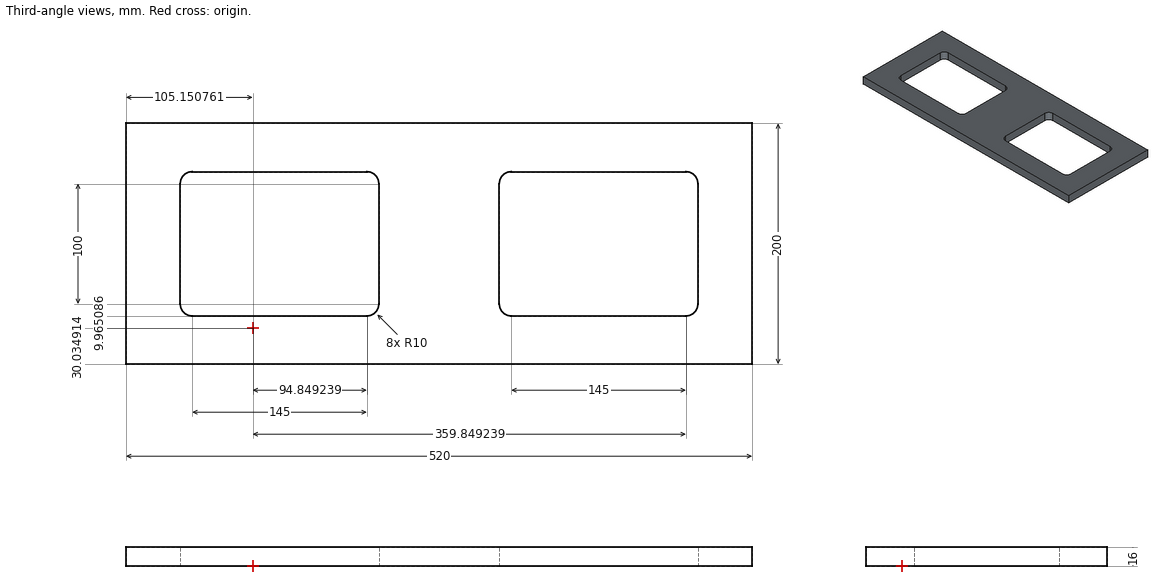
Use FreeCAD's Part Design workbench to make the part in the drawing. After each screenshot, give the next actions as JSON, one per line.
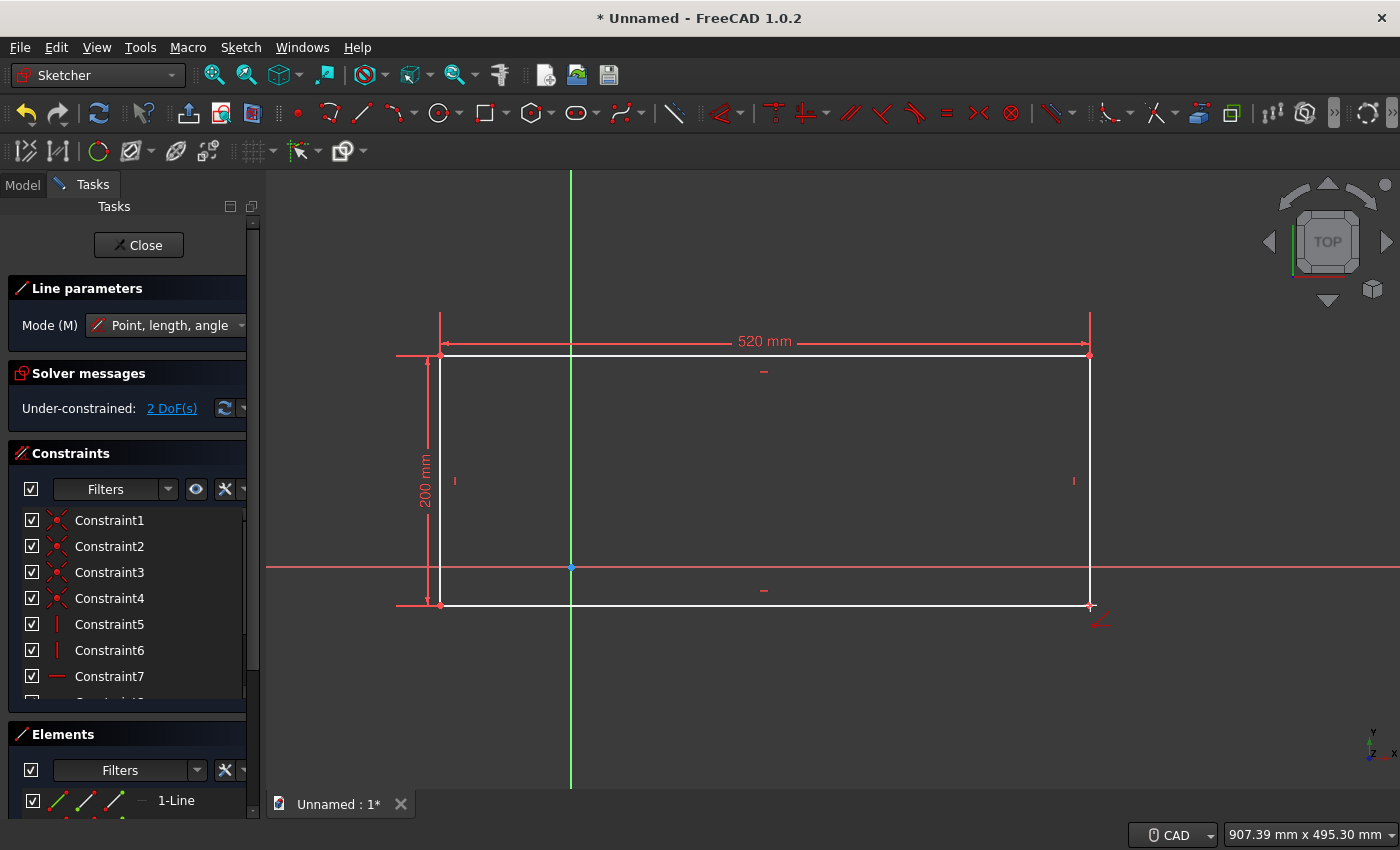
{"action": "left_click", "coordinate": [702, 417]}
{"action": "left_click", "coordinate": [702, 542]}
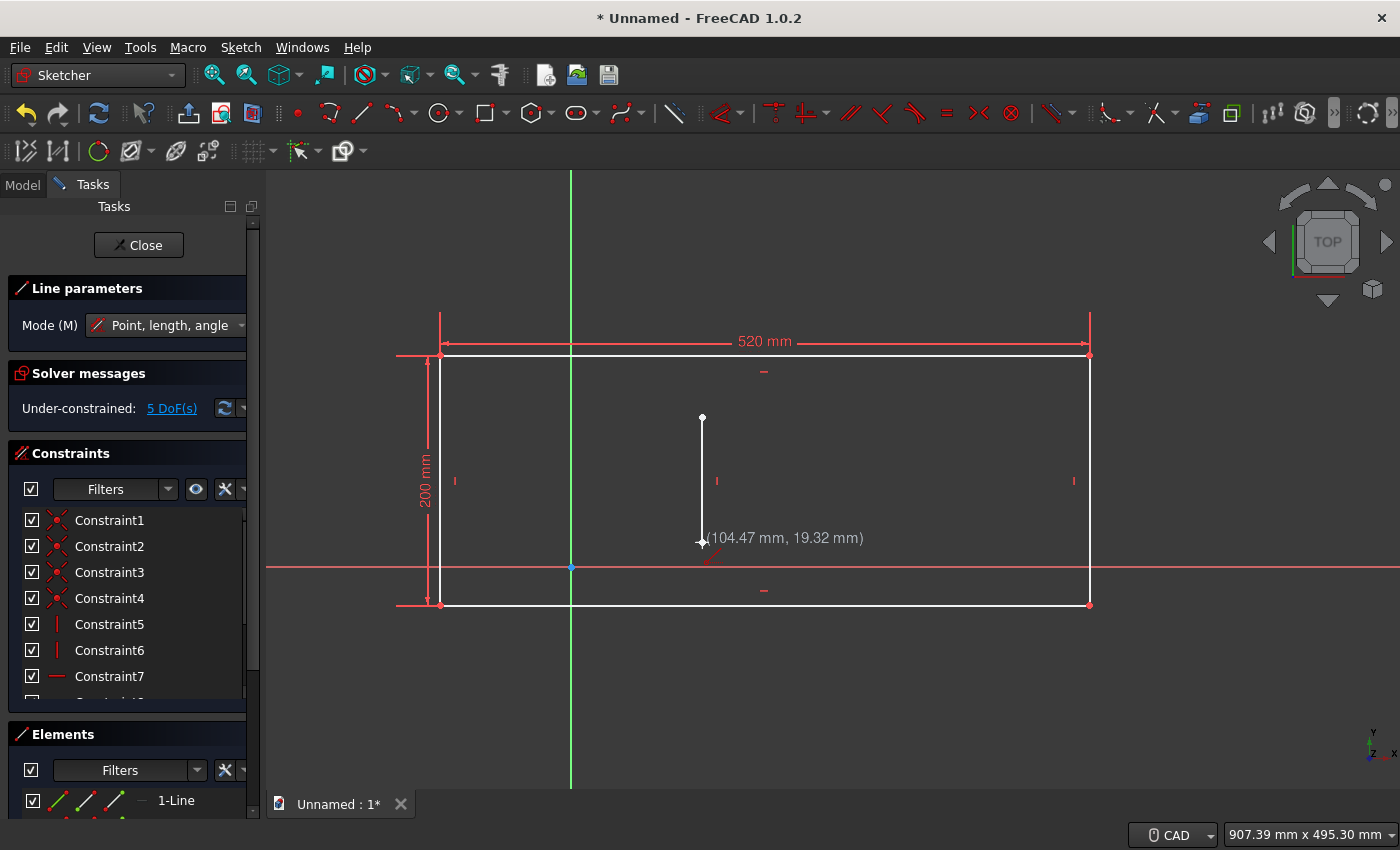
{"action": "scroll", "coordinate": [690, 555], "scroll_direction": "up", "scroll_amount": 2}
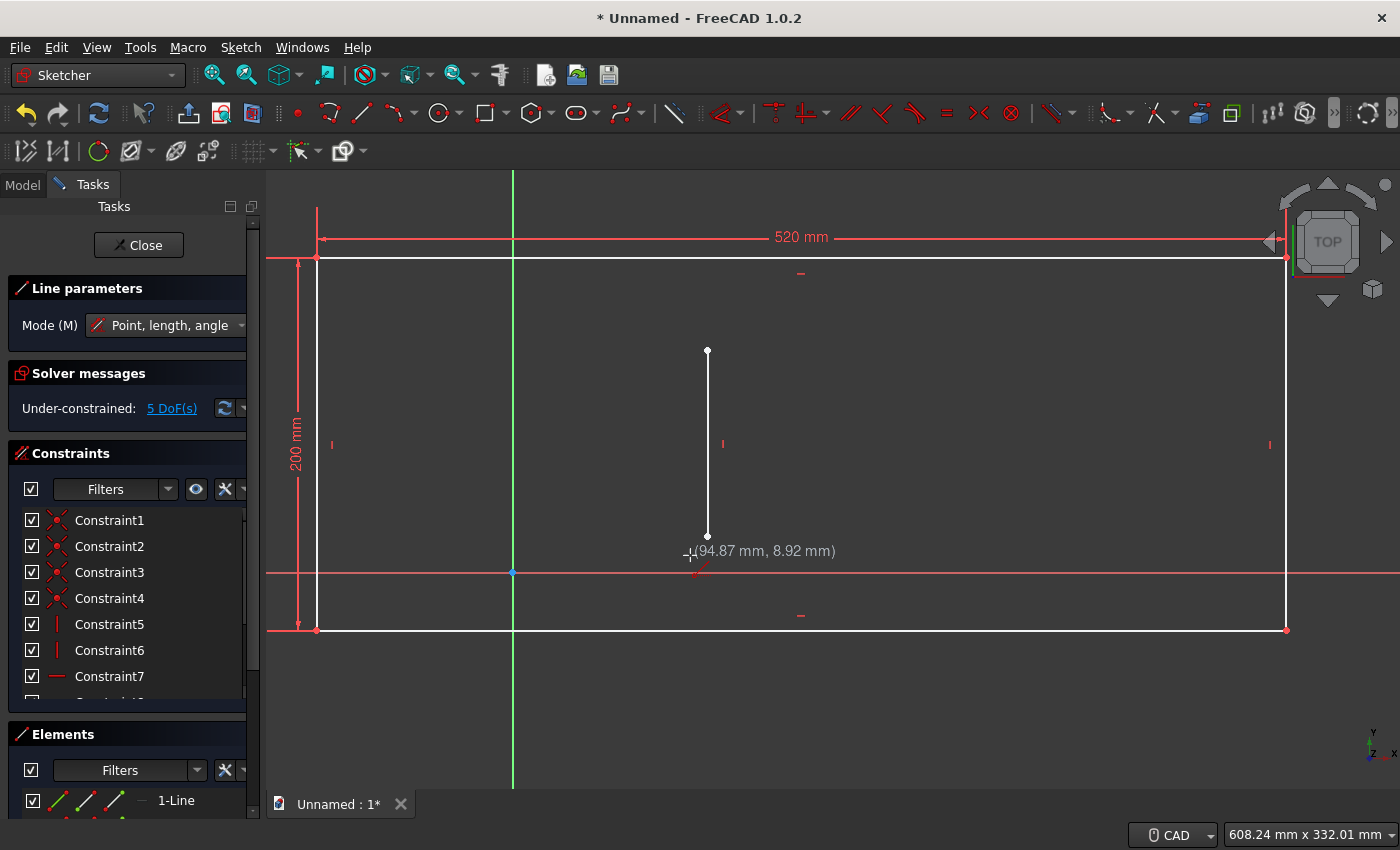
{"action": "left_click", "coordinate": [690, 554]}
{"action": "left_click", "coordinate": [419, 554]}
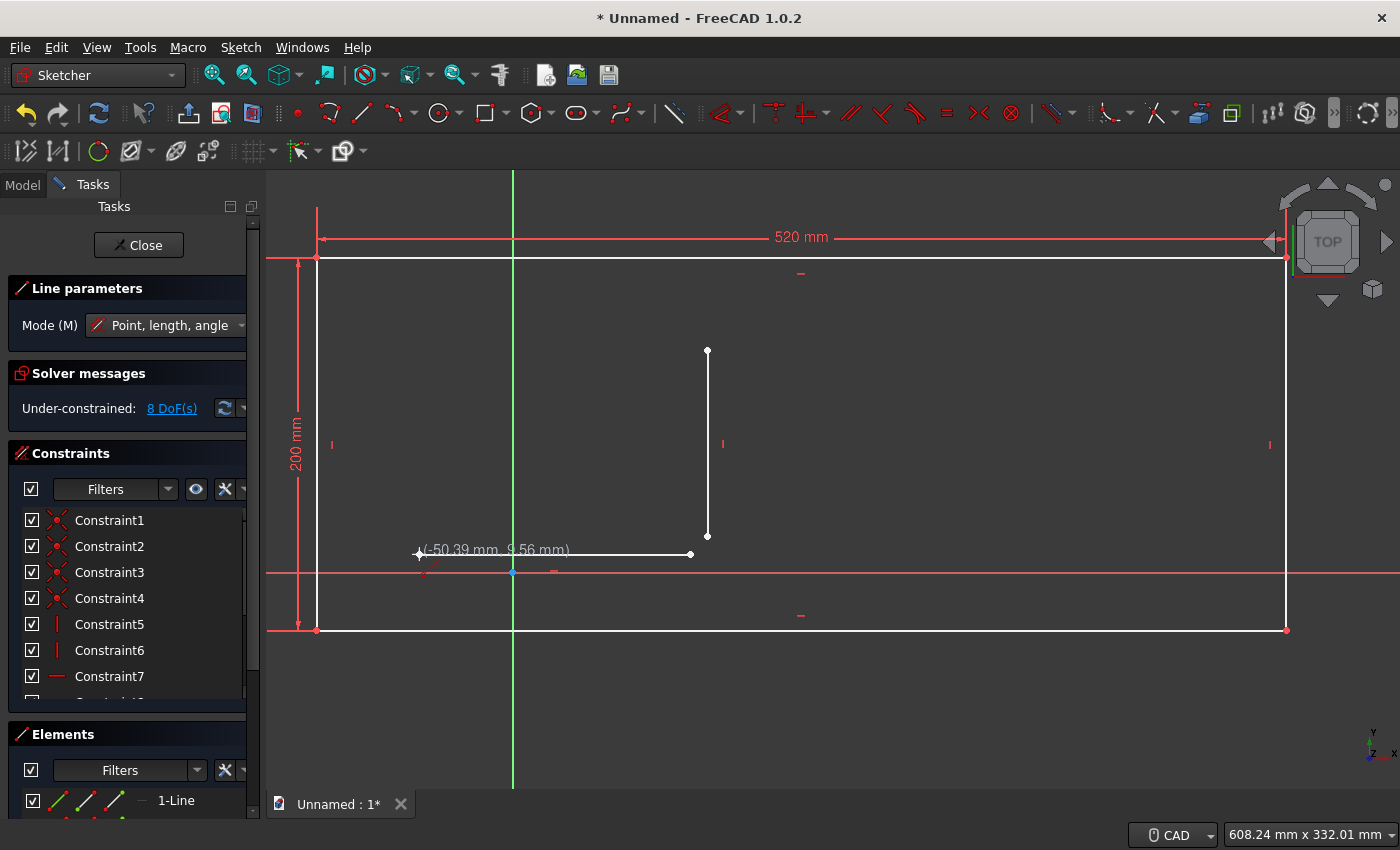
{"action": "left_click", "coordinate": [401, 536]}
{"action": "left_click", "coordinate": [401, 349]}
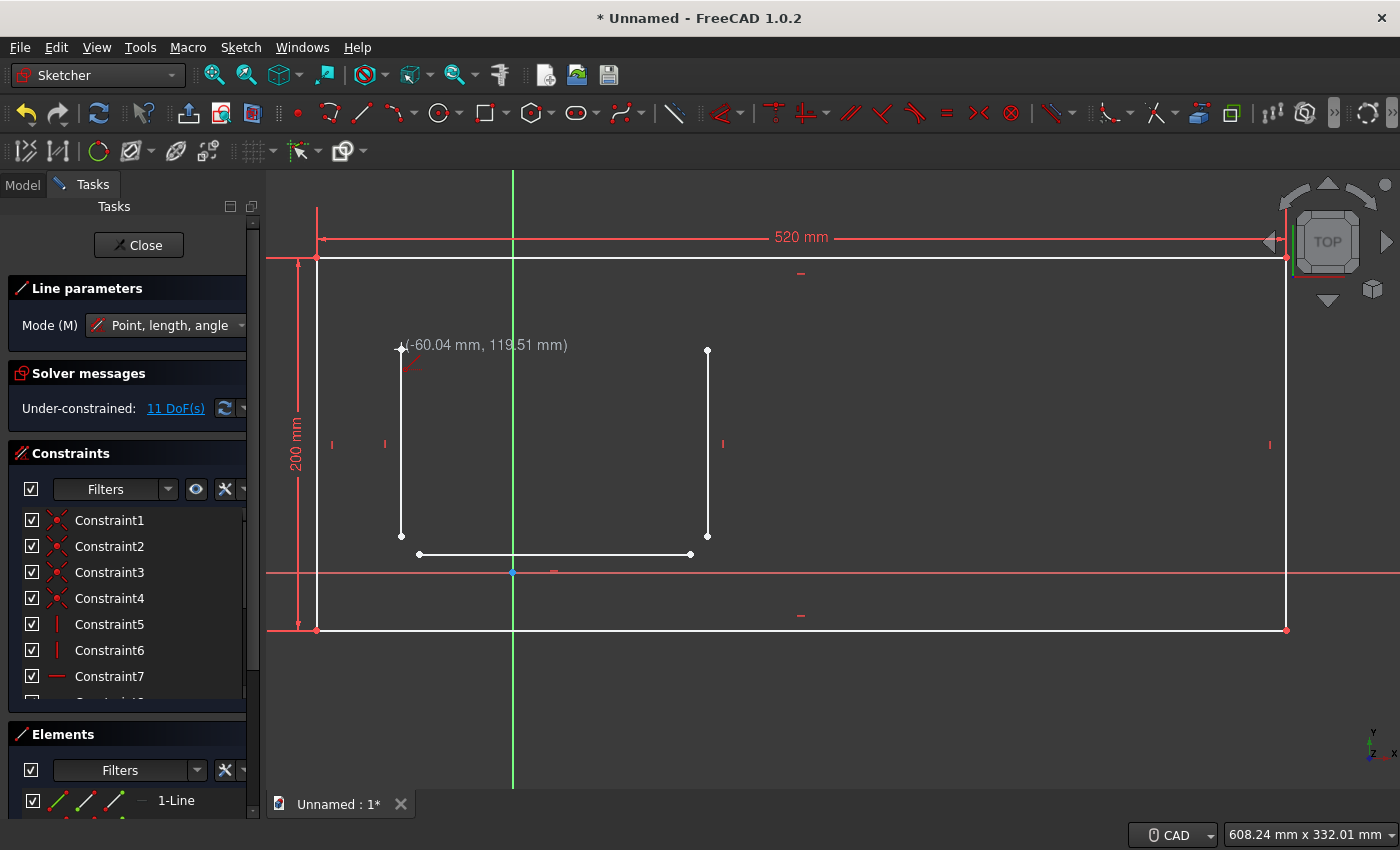
{"action": "left_click", "coordinate": [419, 331]}
{"action": "left_click", "coordinate": [690, 331]}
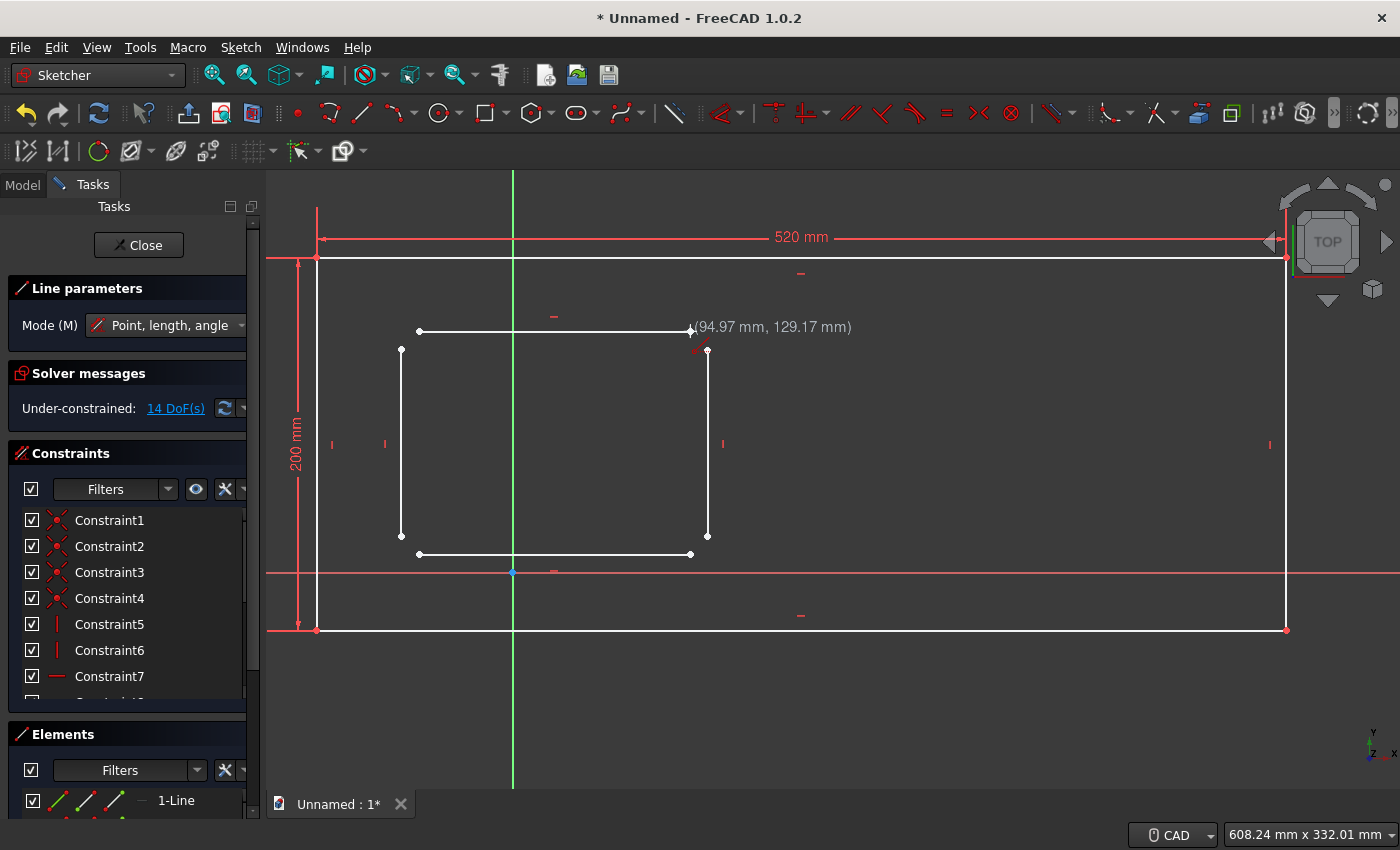
{"action": "key", "text": "g 3 a"}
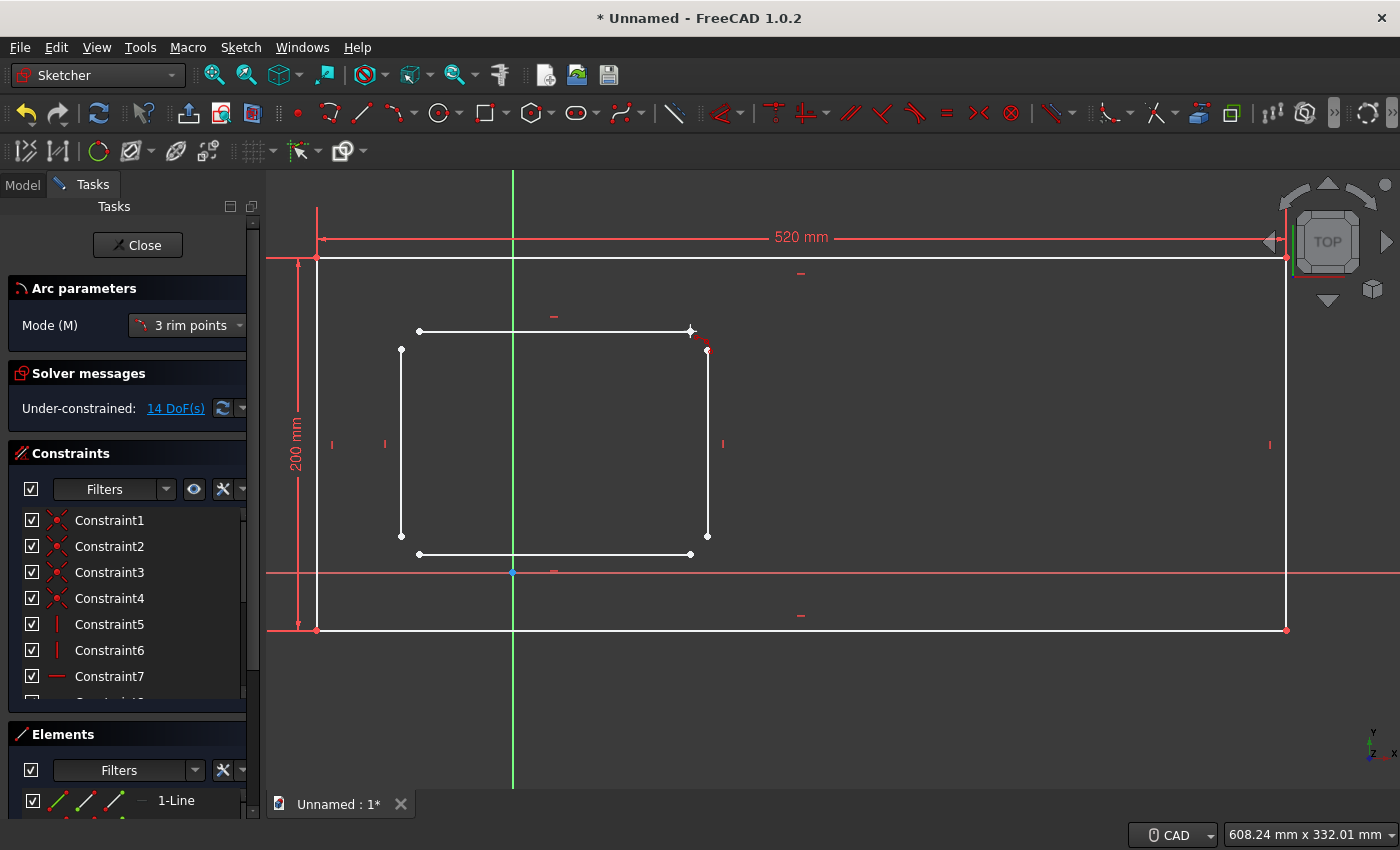
{"action": "left_click", "coordinate": [708, 537]}
{"action": "left_click", "coordinate": [690, 555]}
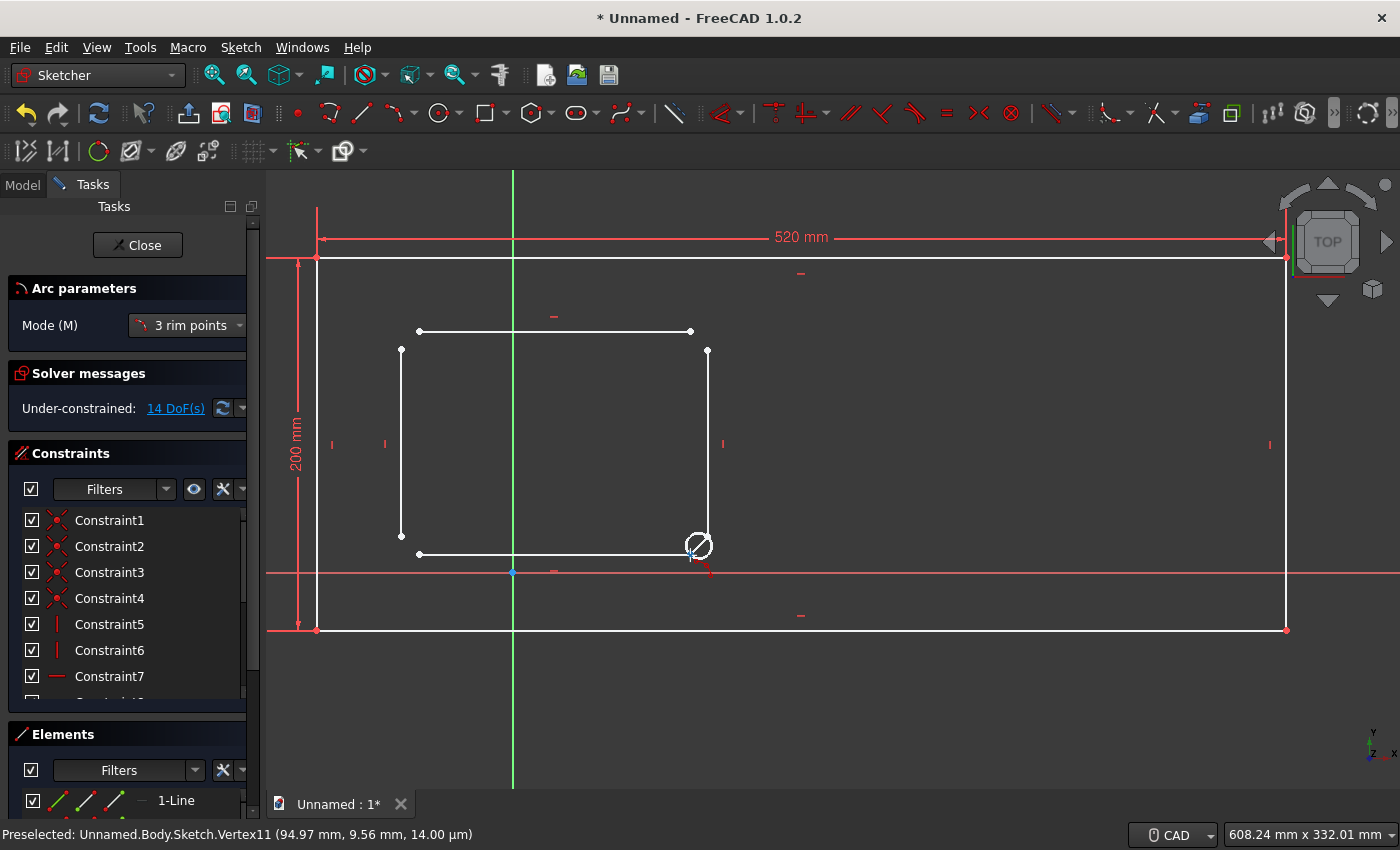
{"action": "scroll", "coordinate": [703, 549], "scroll_direction": "up", "scroll_amount": 6}